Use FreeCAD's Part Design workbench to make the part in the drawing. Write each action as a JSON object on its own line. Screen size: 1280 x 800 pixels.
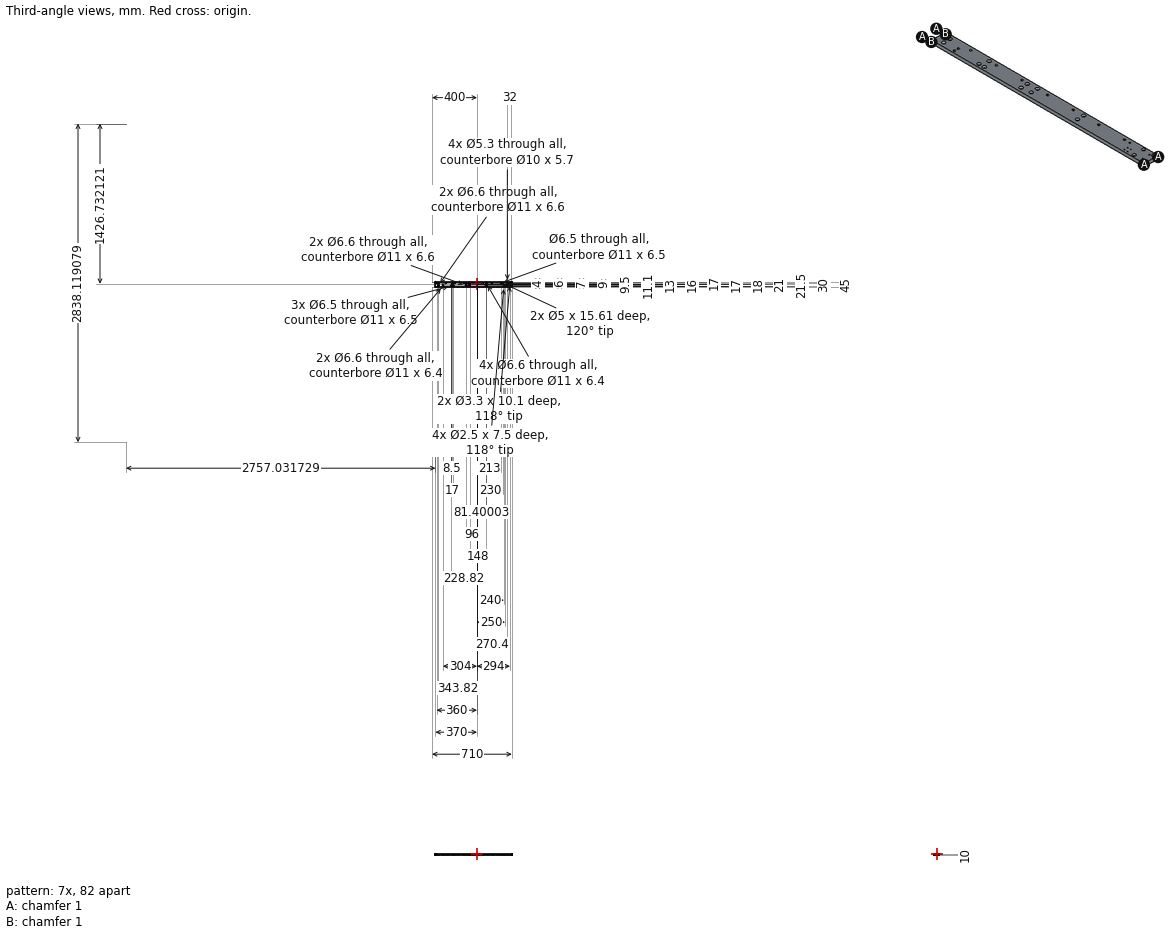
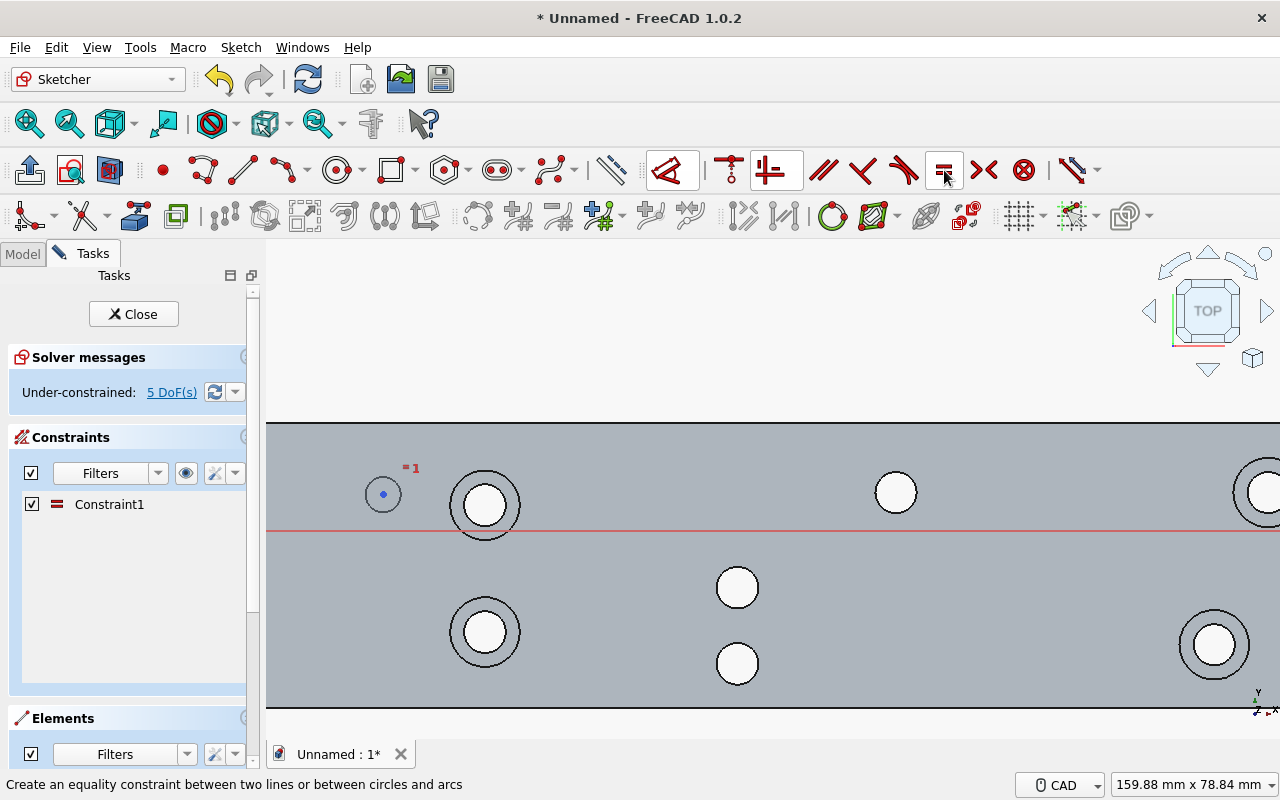
{"action": "scroll", "coordinate": [398, 486], "scroll_direction": "down", "scroll_amount": 9}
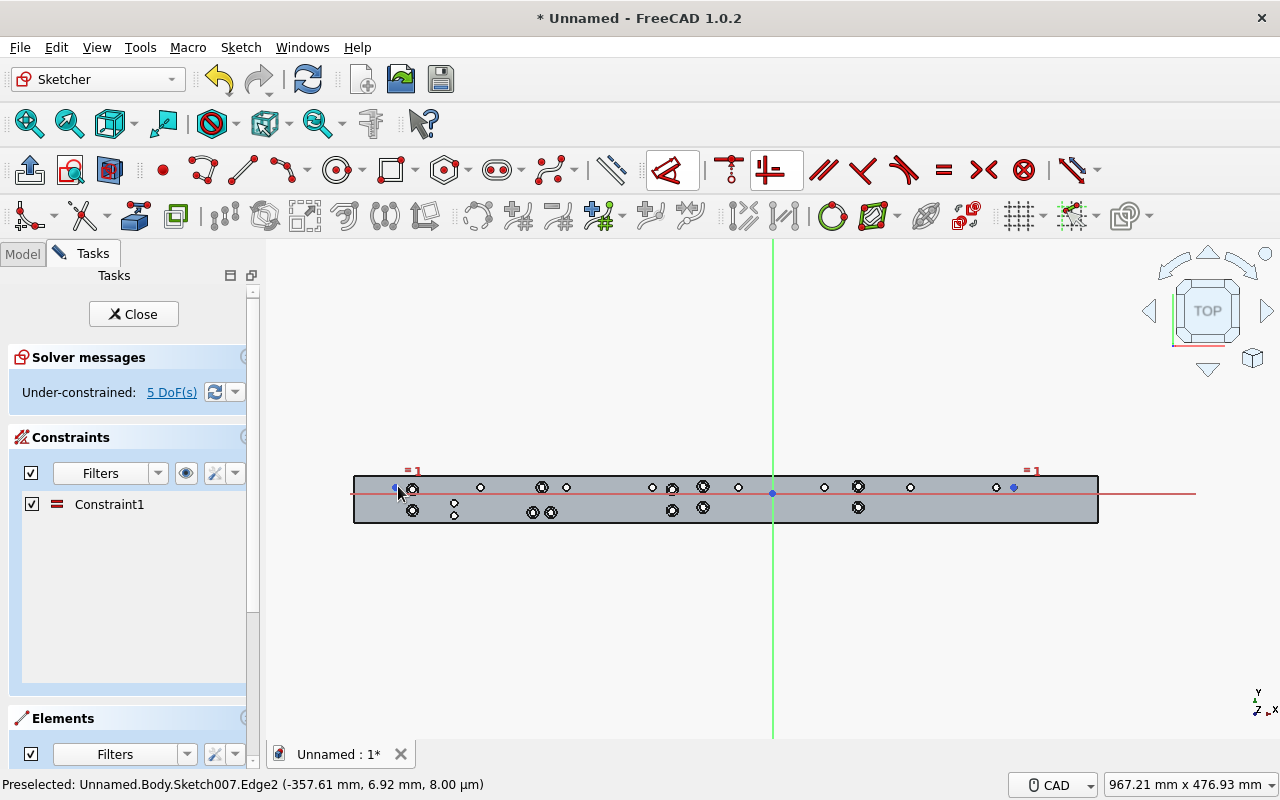
{"action": "left_click", "coordinate": [1014, 488]}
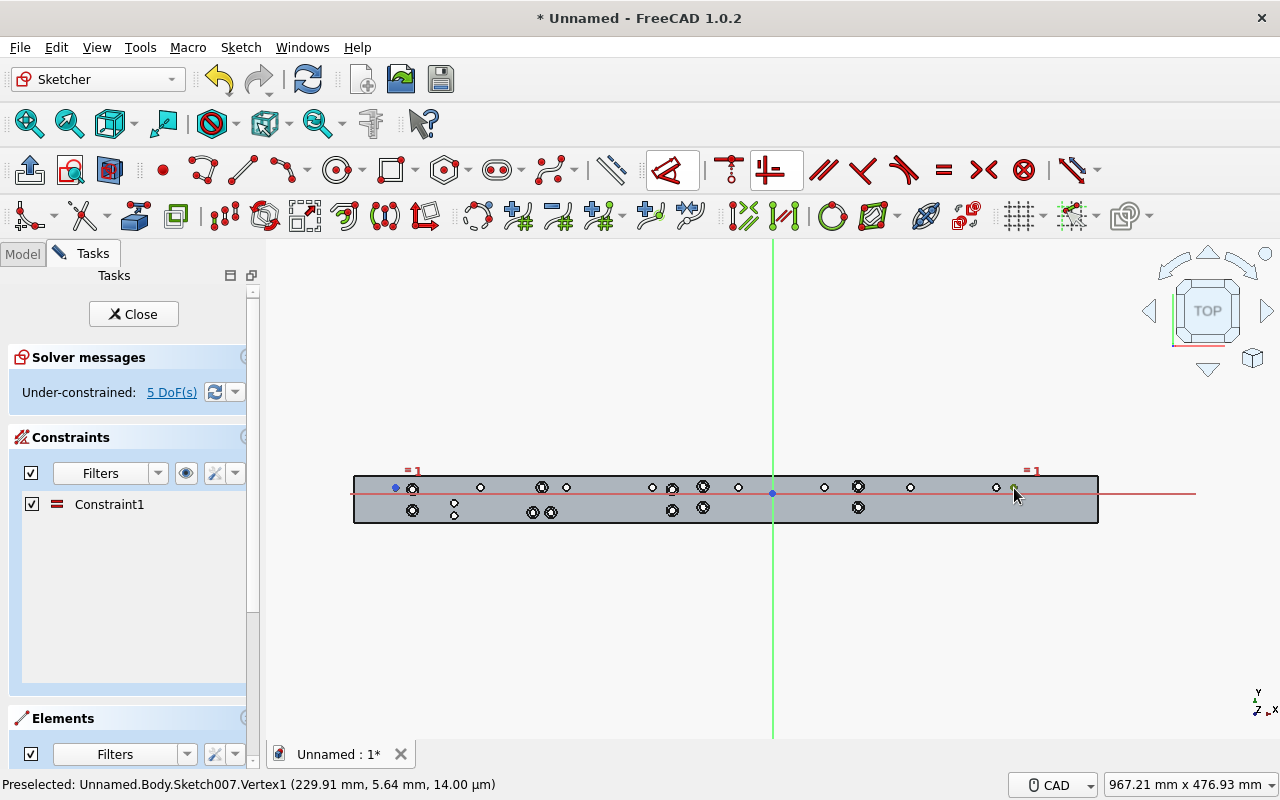
{"action": "left_click", "coordinate": [396, 488]}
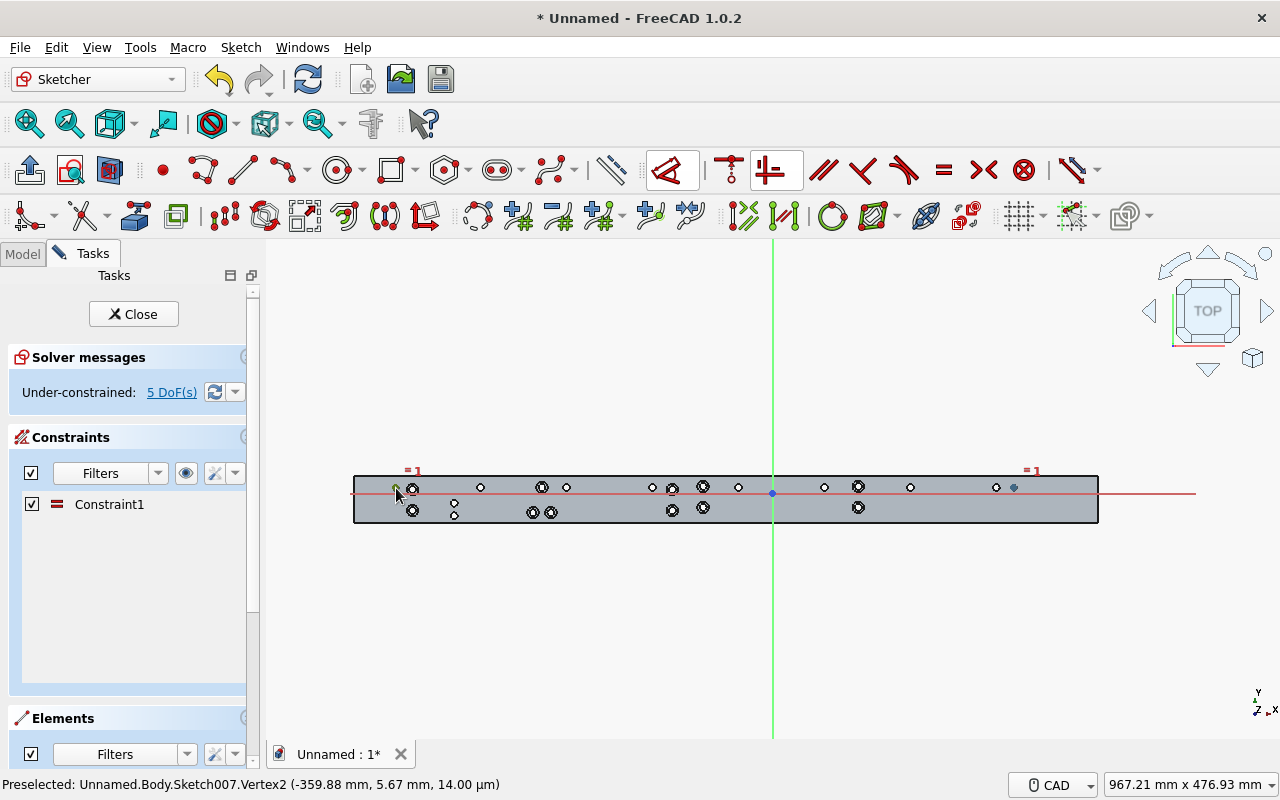
{"action": "left_click", "coordinate": [798, 170]}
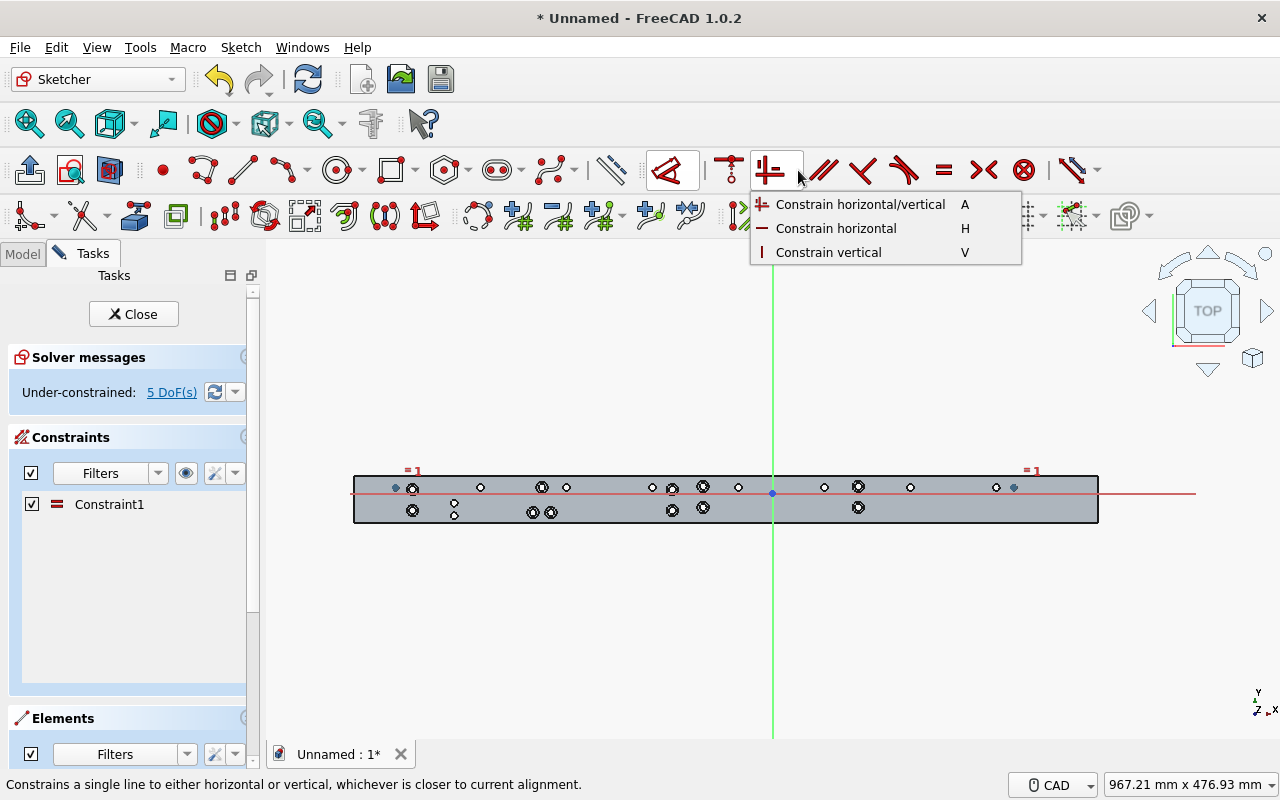
{"action": "left_click", "coordinate": [886, 228]}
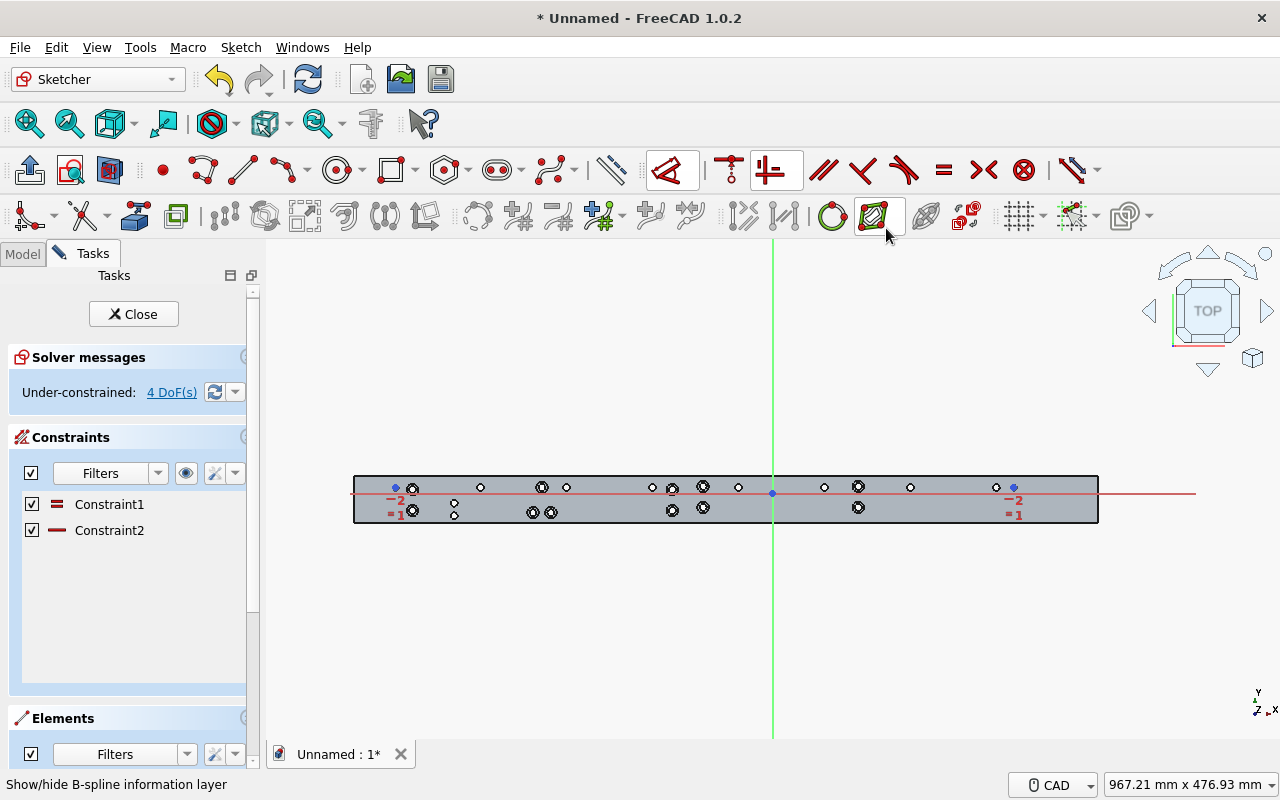
{"action": "scroll", "coordinate": [1014, 491], "scroll_direction": "up", "scroll_amount": 11}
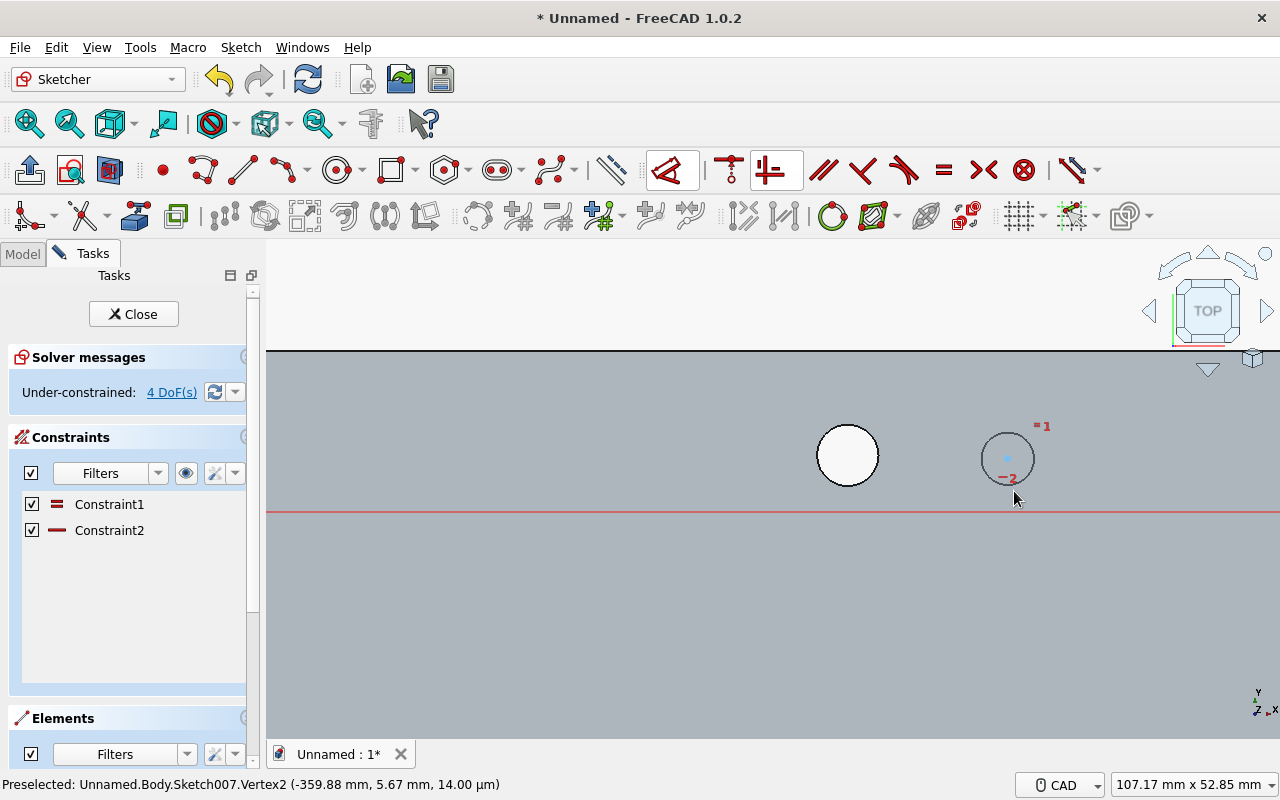
{"action": "left_click", "coordinate": [1009, 433]}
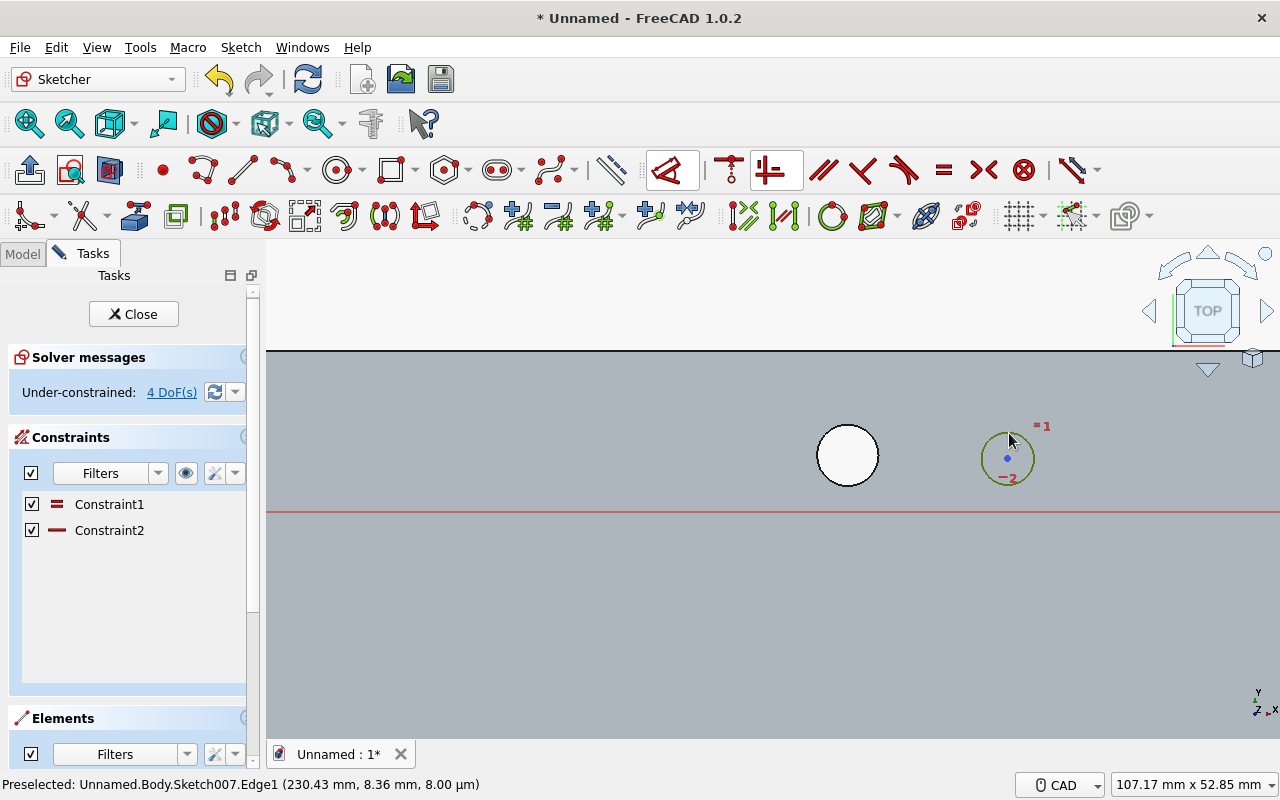
{"action": "left_click", "coordinate": [694, 170]}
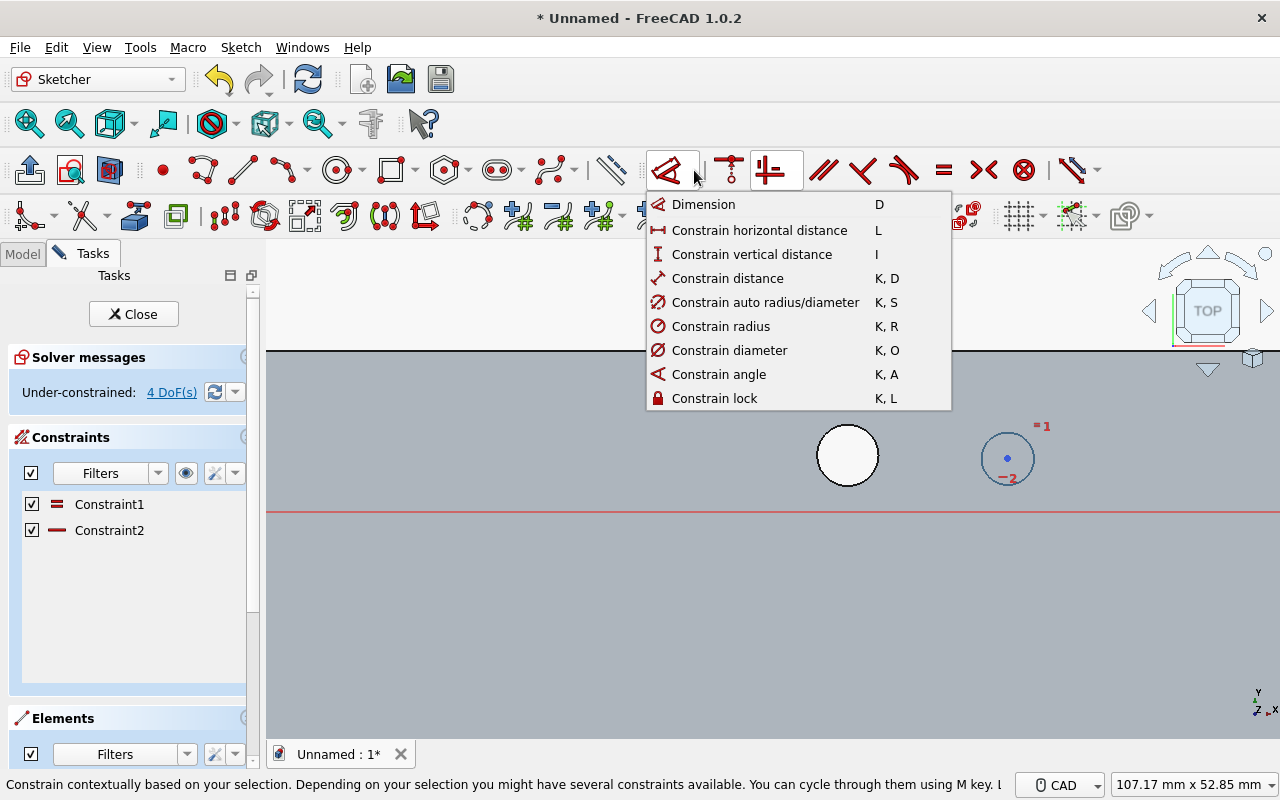
{"action": "left_click", "coordinate": [799, 350]}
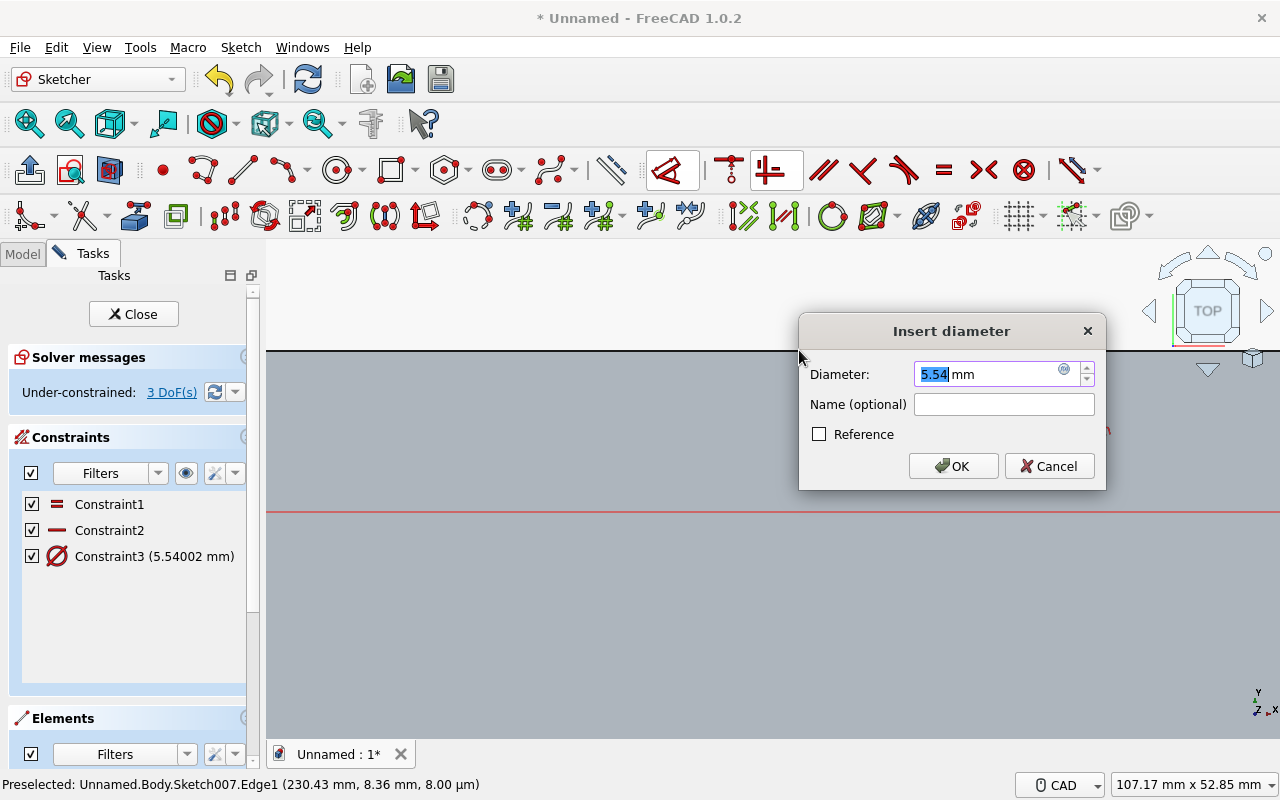
{"action": "type", "text": "5"}
{"action": "key", "text": "Return"}